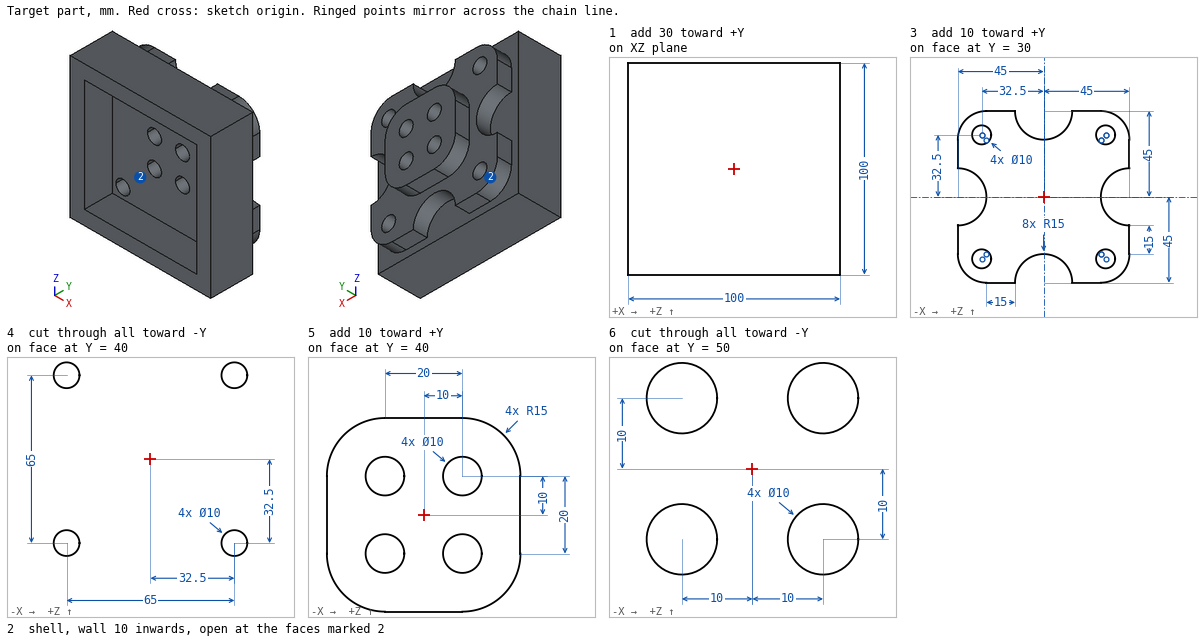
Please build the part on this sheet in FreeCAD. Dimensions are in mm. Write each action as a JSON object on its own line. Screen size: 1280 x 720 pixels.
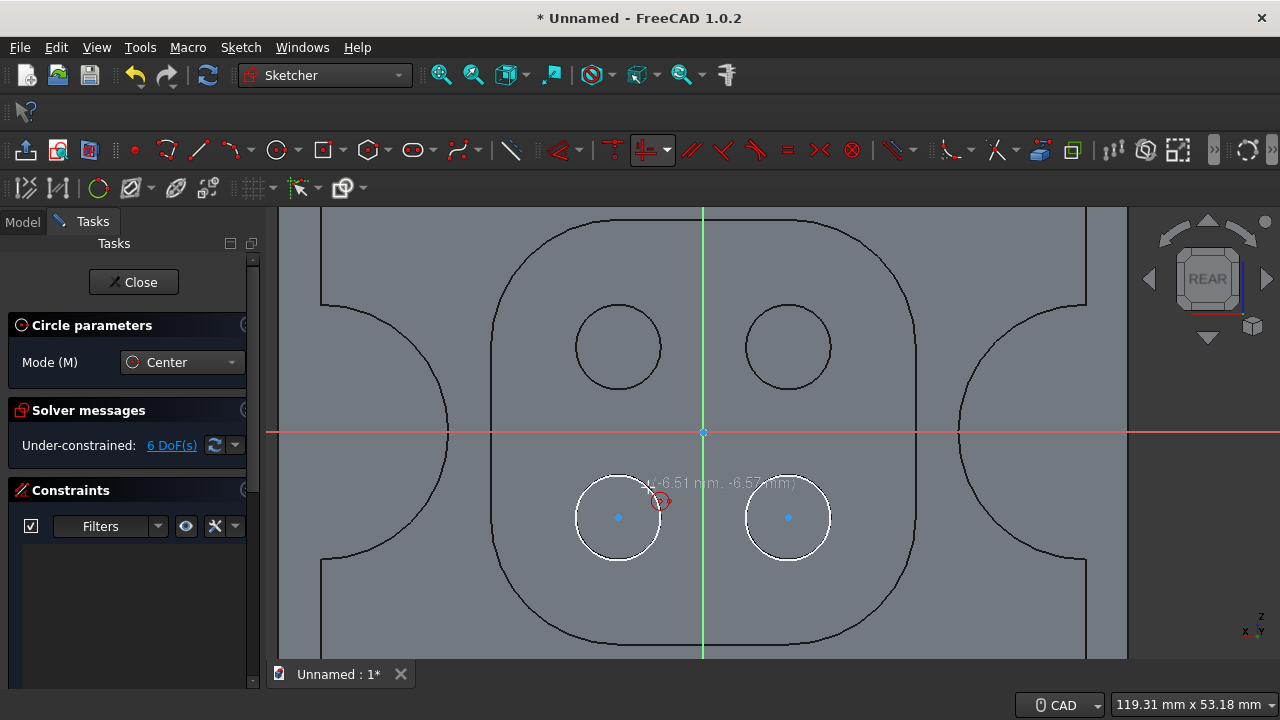
{"action": "left_click", "coordinate": [618, 347]}
{"action": "left_click", "coordinate": [648, 317]}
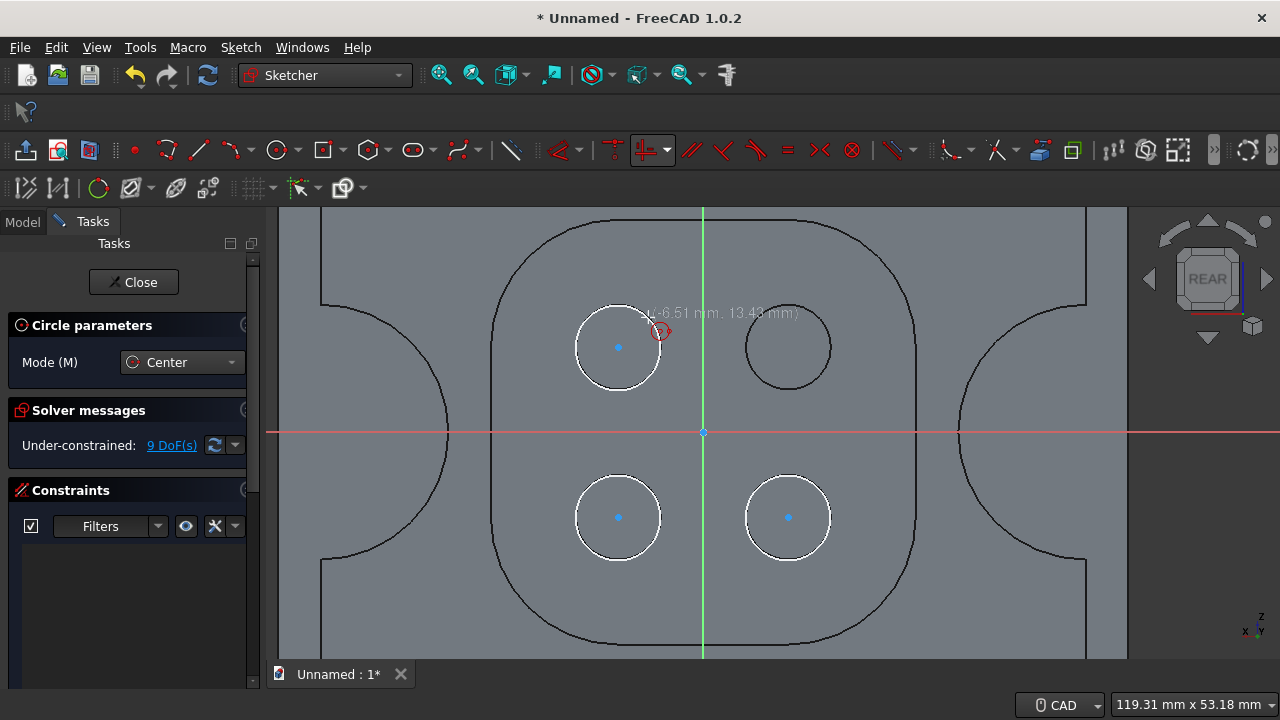
{"action": "left_click", "coordinate": [788, 347]}
{"action": "left_click", "coordinate": [818, 317]}
{"action": "key", "text": "Escape"}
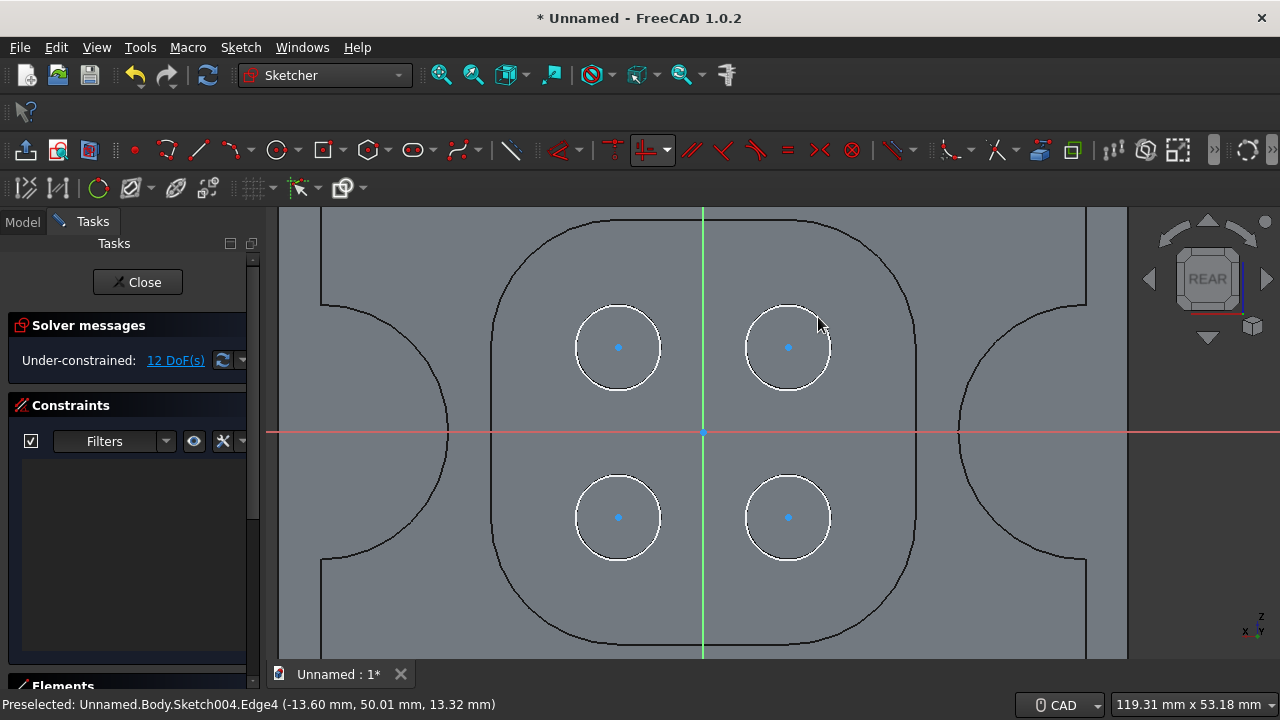
{"action": "left_click", "coordinate": [818, 488]}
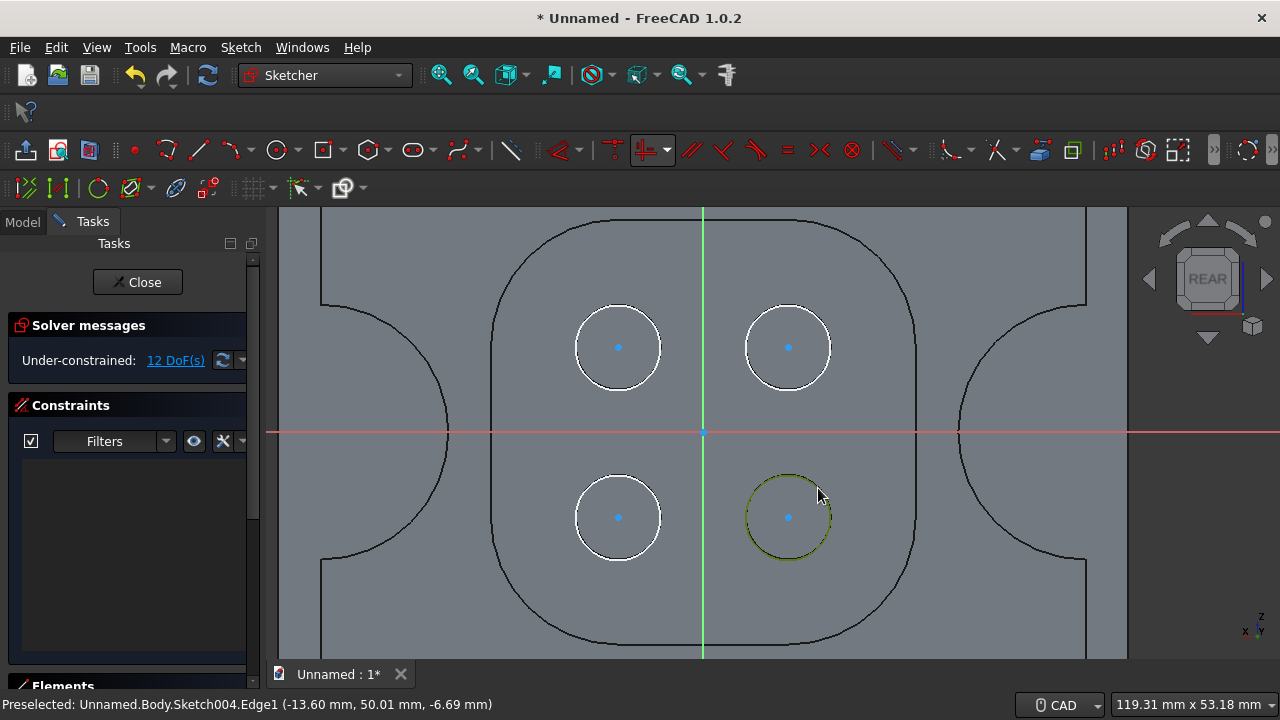
{"action": "left_click", "coordinate": [648, 488]}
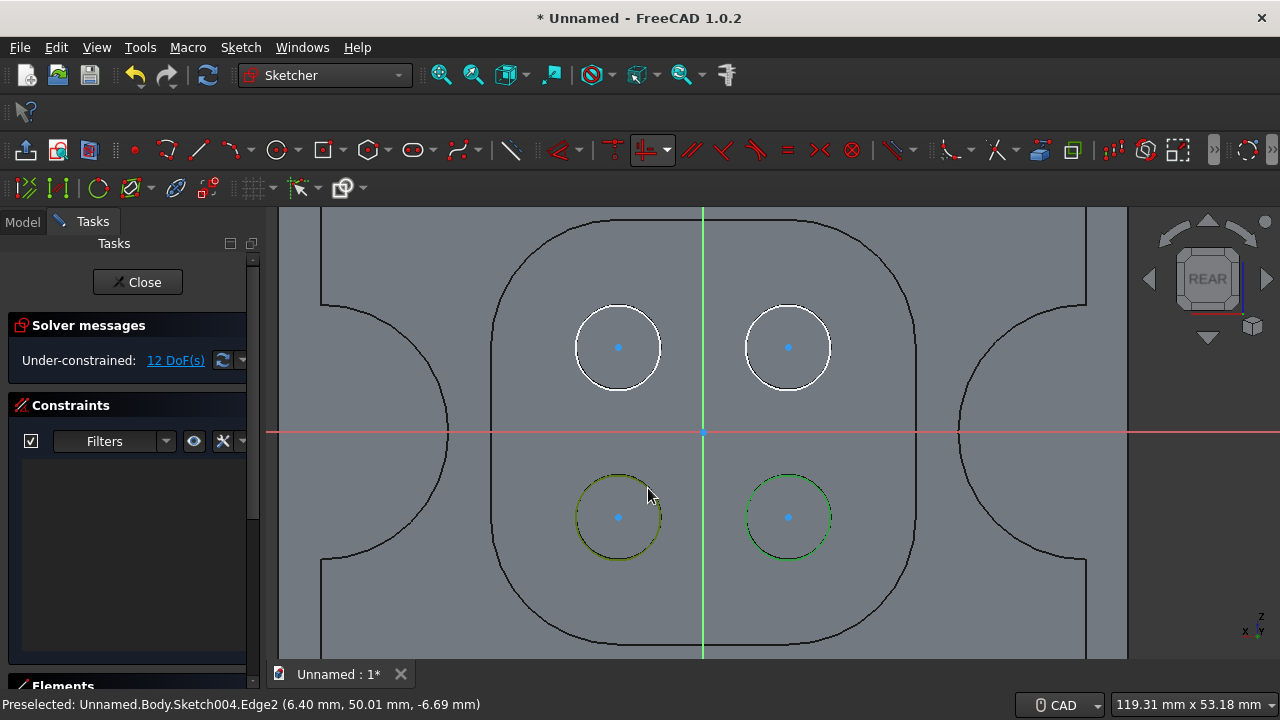
{"action": "left_click", "coordinate": [648, 318]}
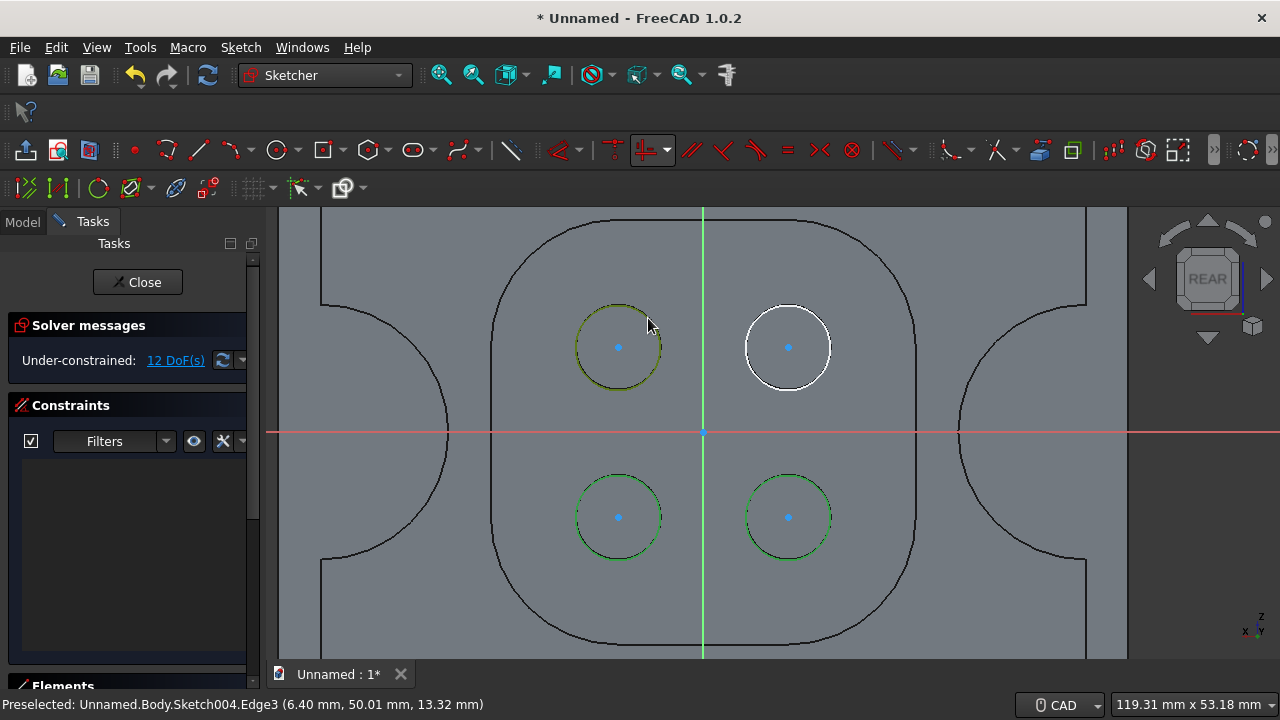
{"action": "left_click", "coordinate": [818, 318]}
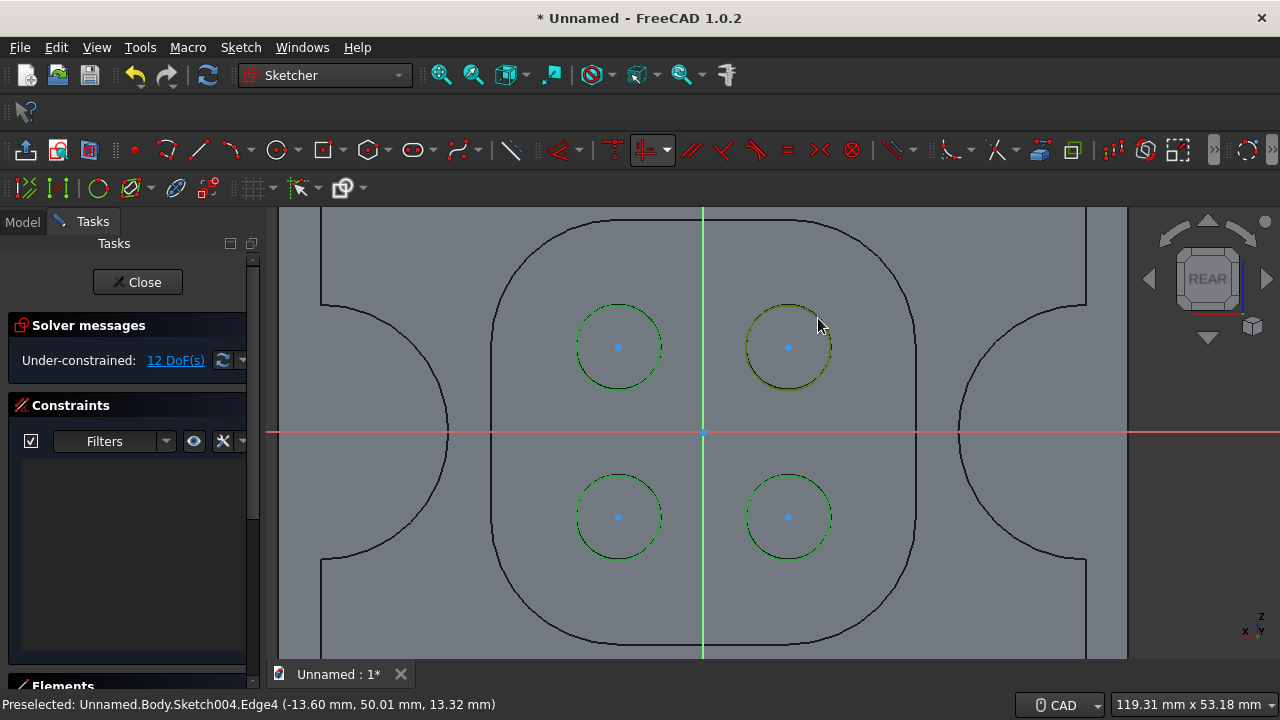
{"action": "left_click", "coordinate": [788, 150]}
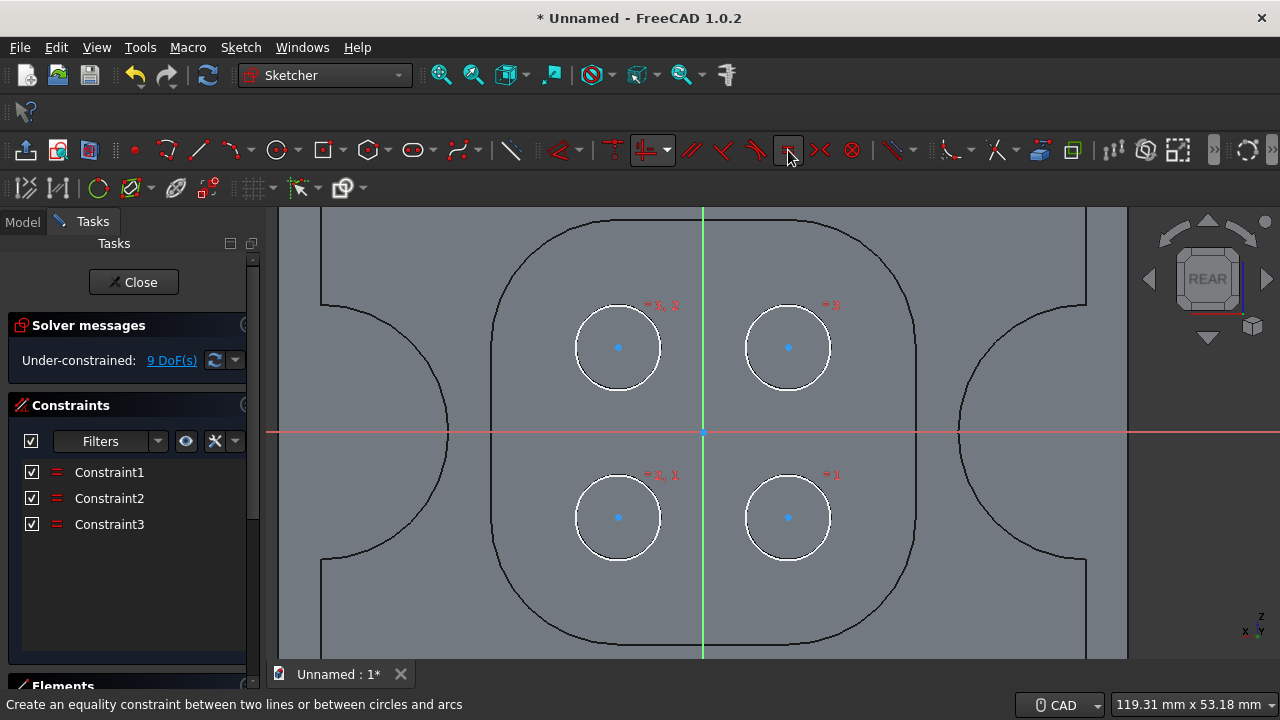
{"action": "left_click", "coordinate": [788, 518]}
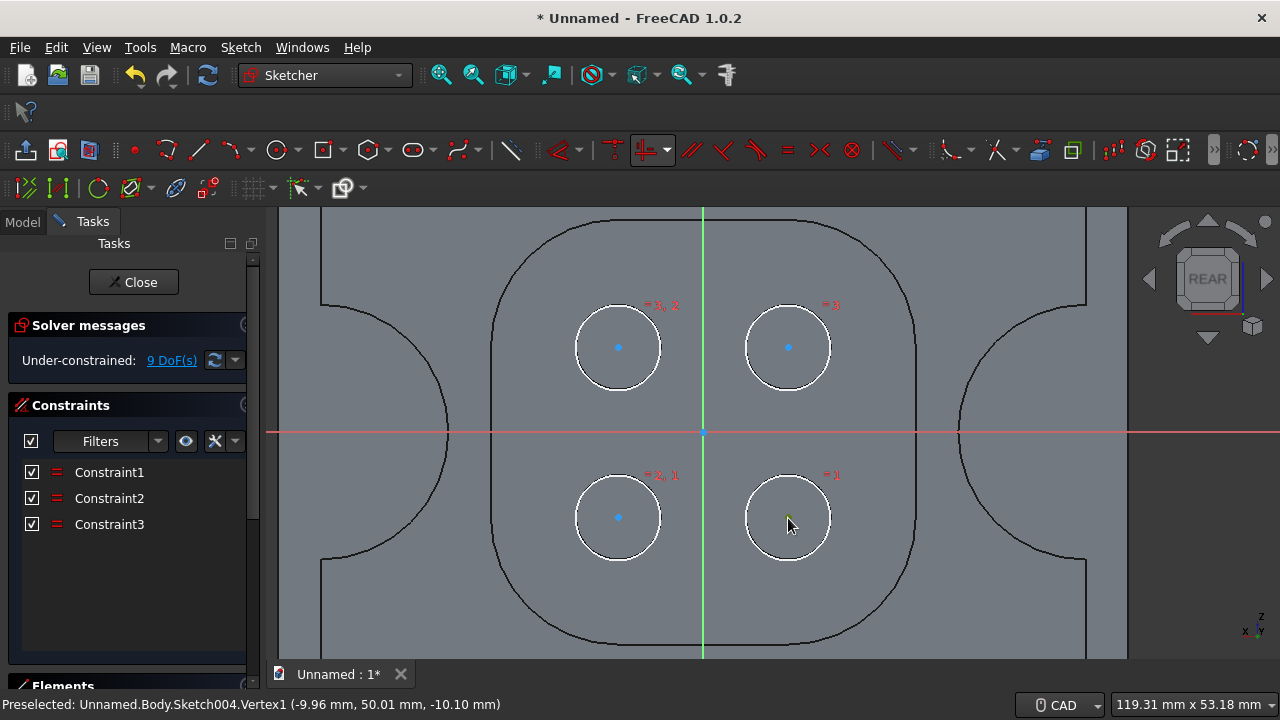
{"action": "left_click", "coordinate": [618, 518]}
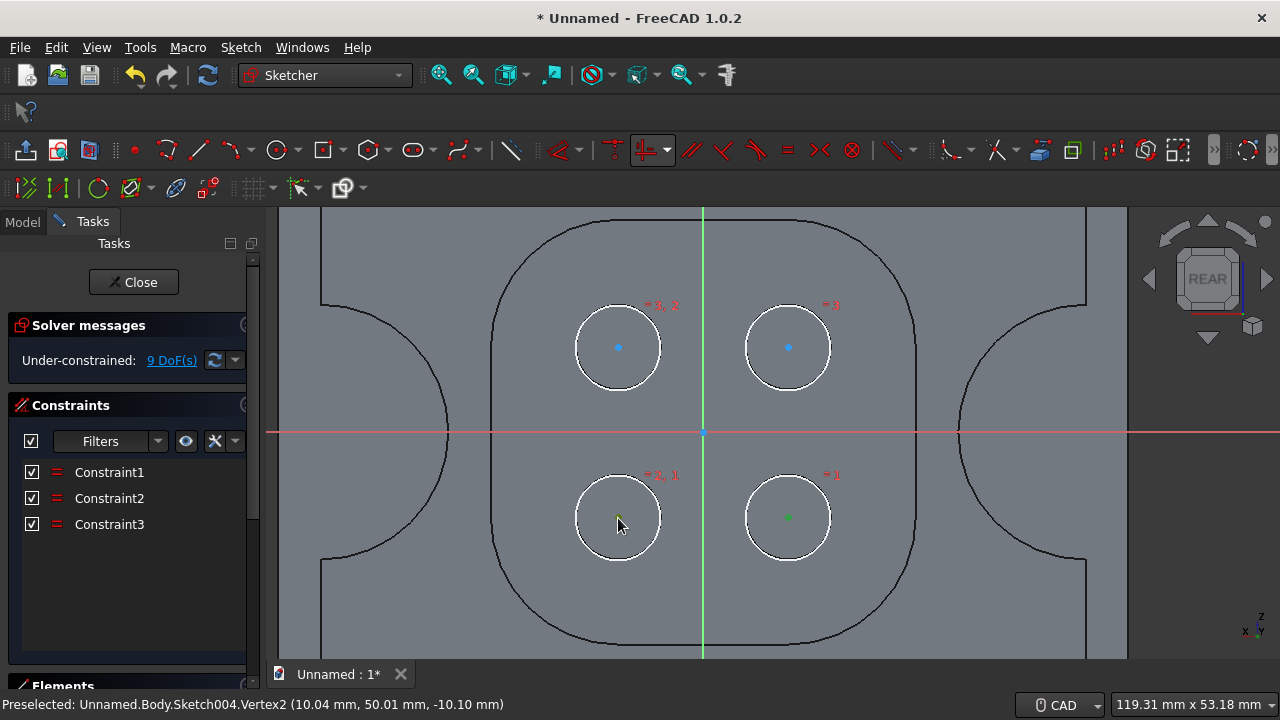
{"action": "left_click", "coordinate": [670, 150]}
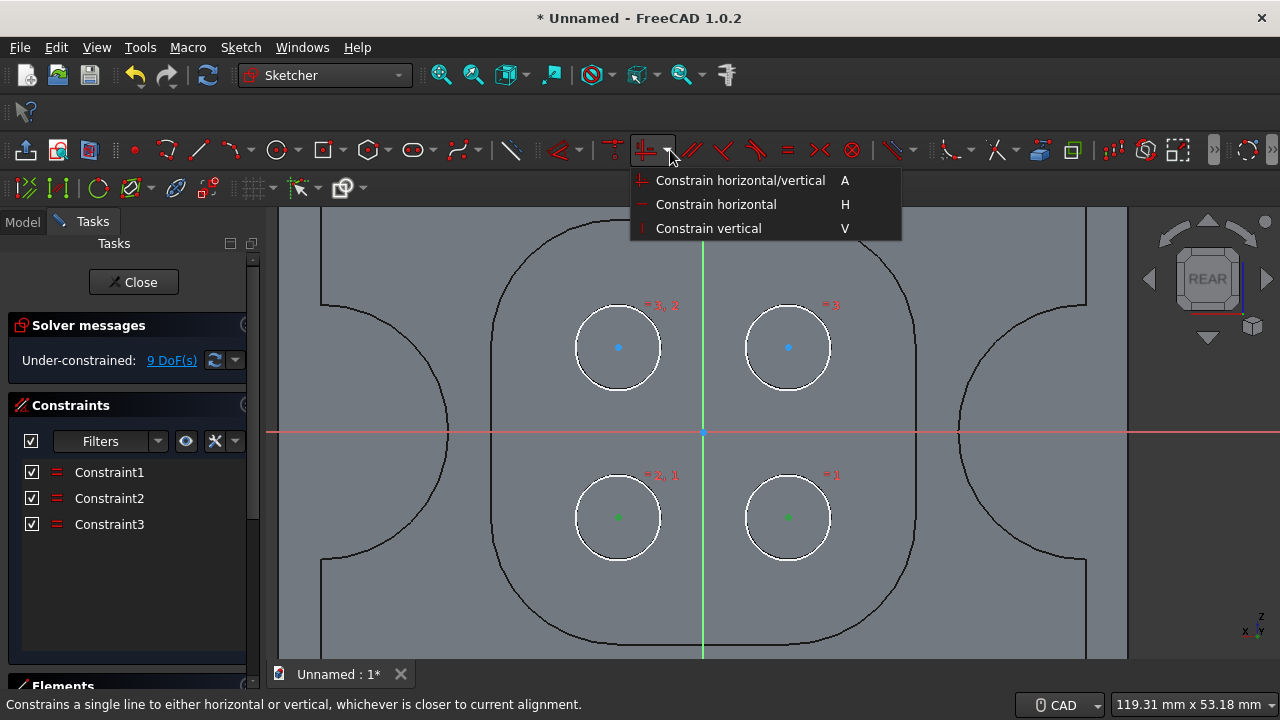
{"action": "left_click", "coordinate": [766, 204]}